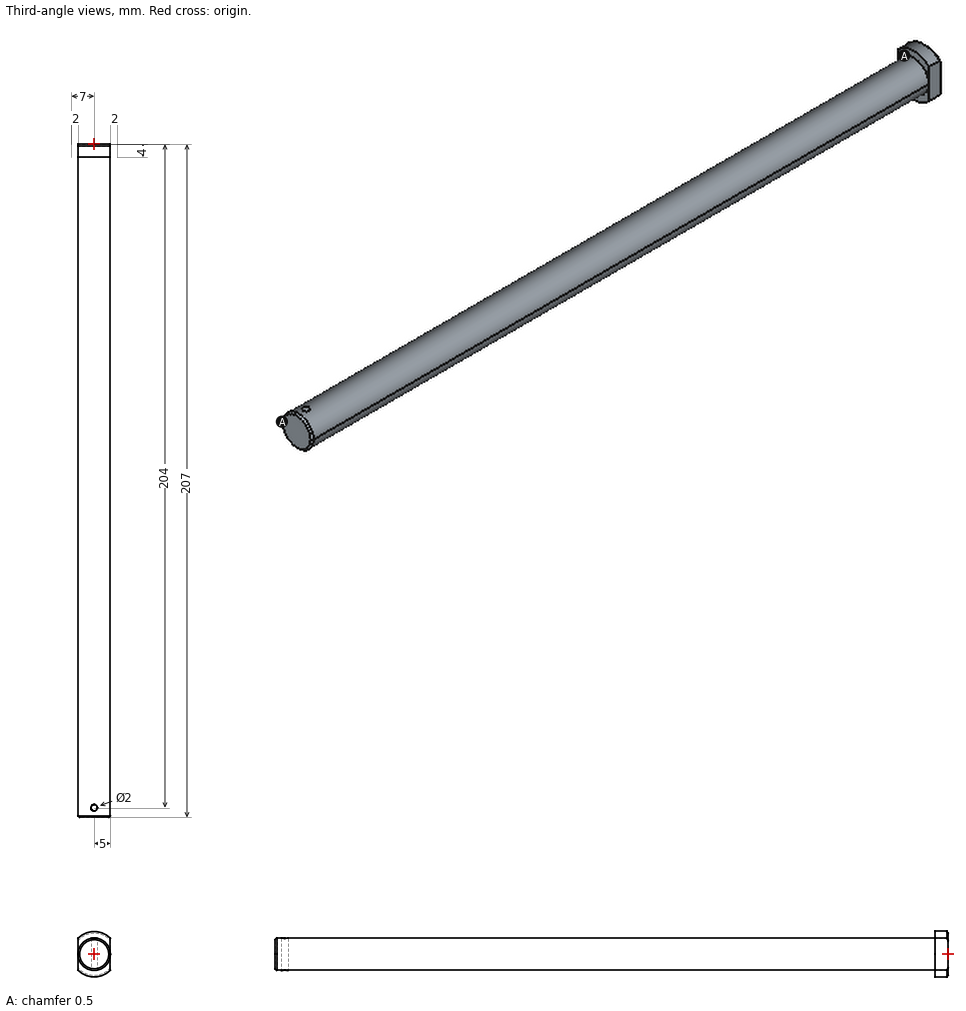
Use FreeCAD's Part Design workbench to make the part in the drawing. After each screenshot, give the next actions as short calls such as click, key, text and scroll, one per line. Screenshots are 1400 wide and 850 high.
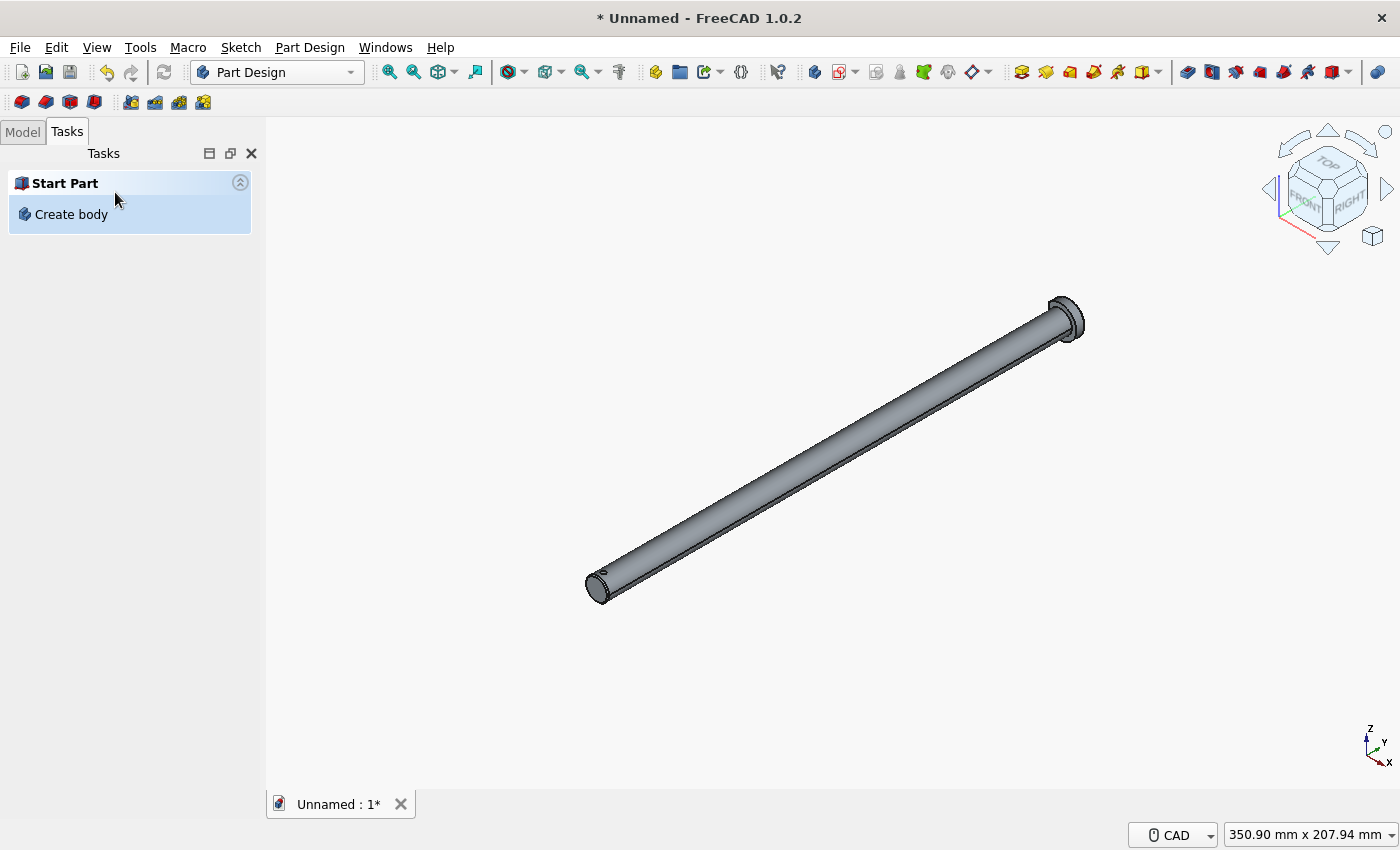
click(840, 72)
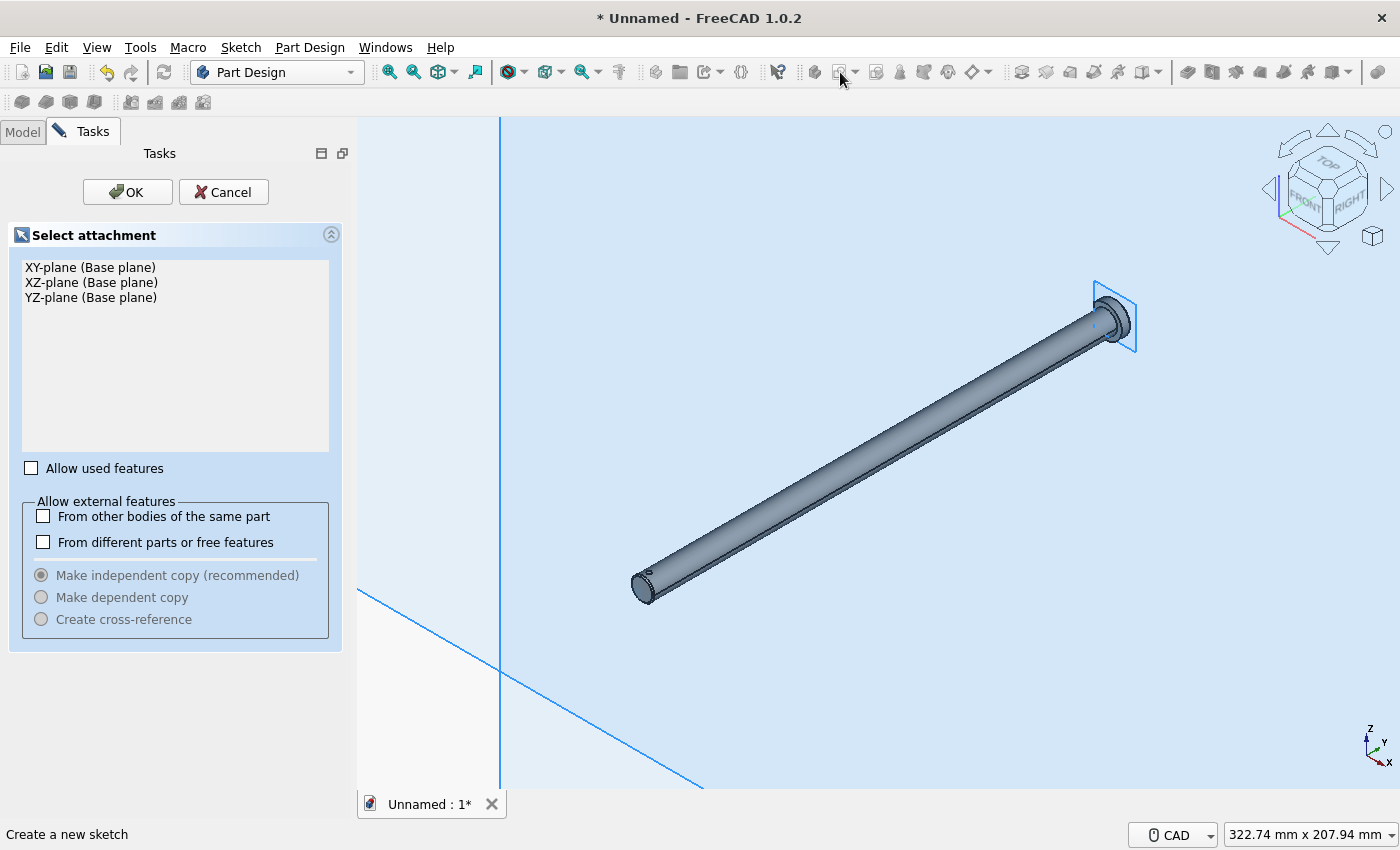
click(82, 268)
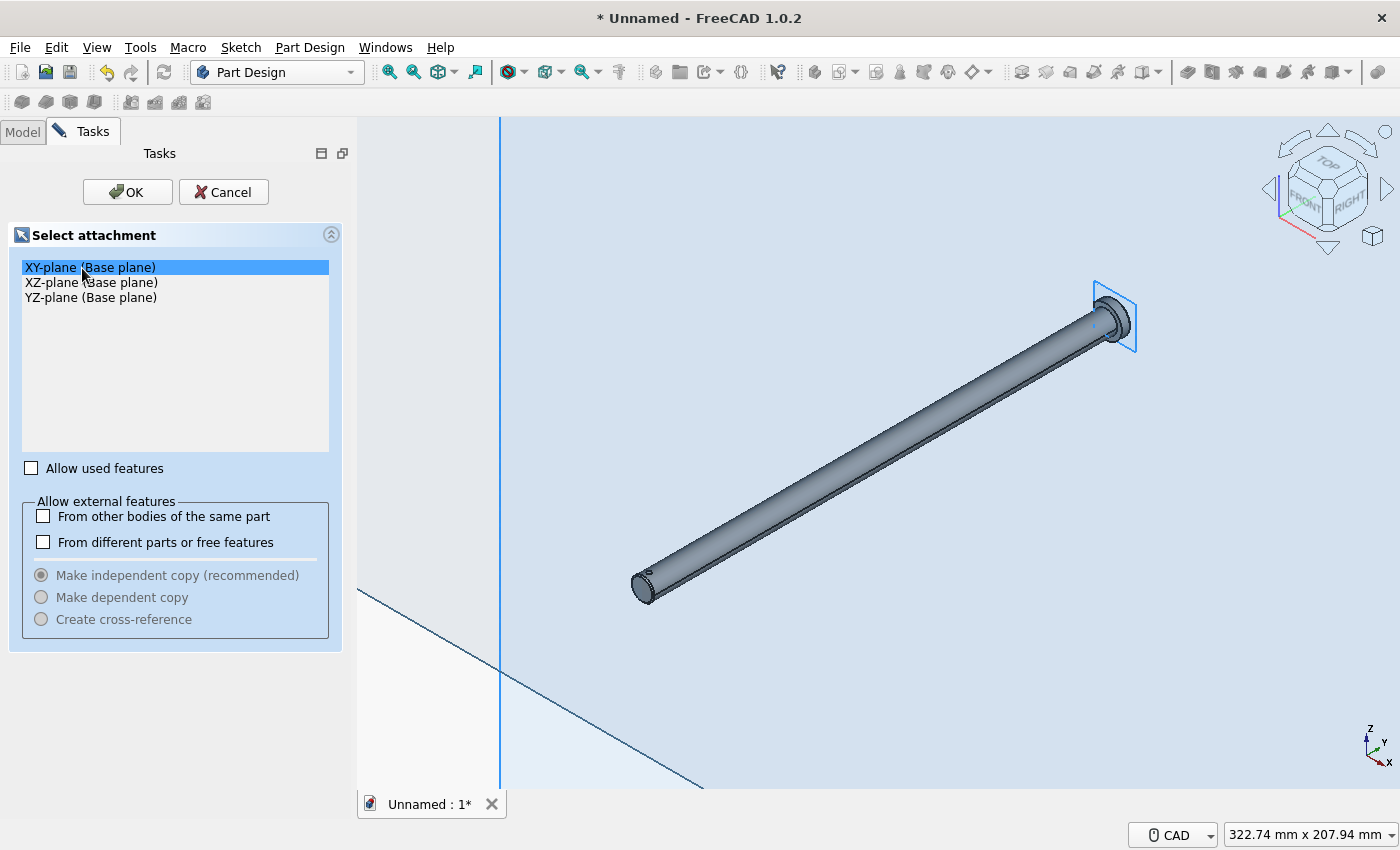
click(128, 192)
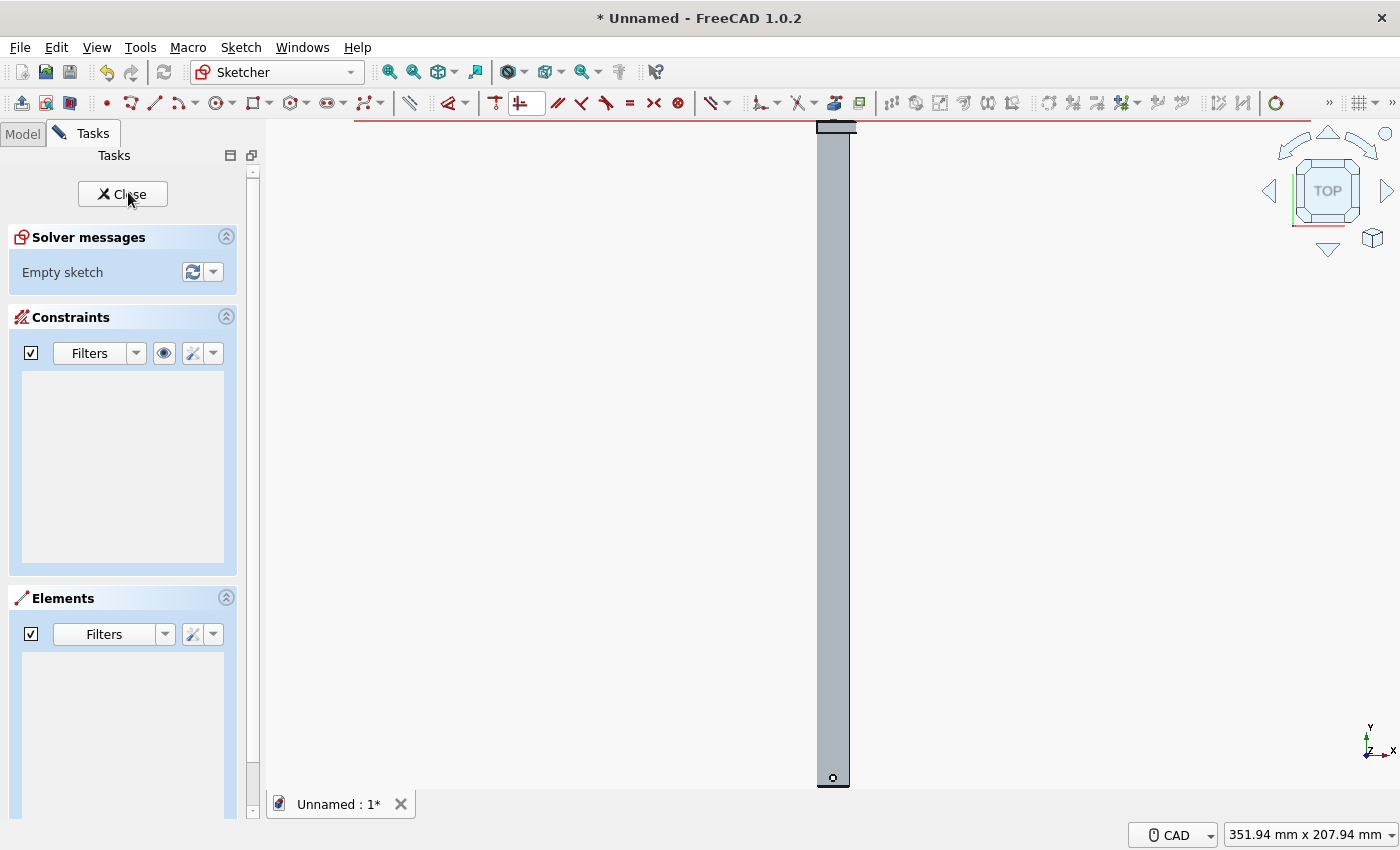
click(70, 104)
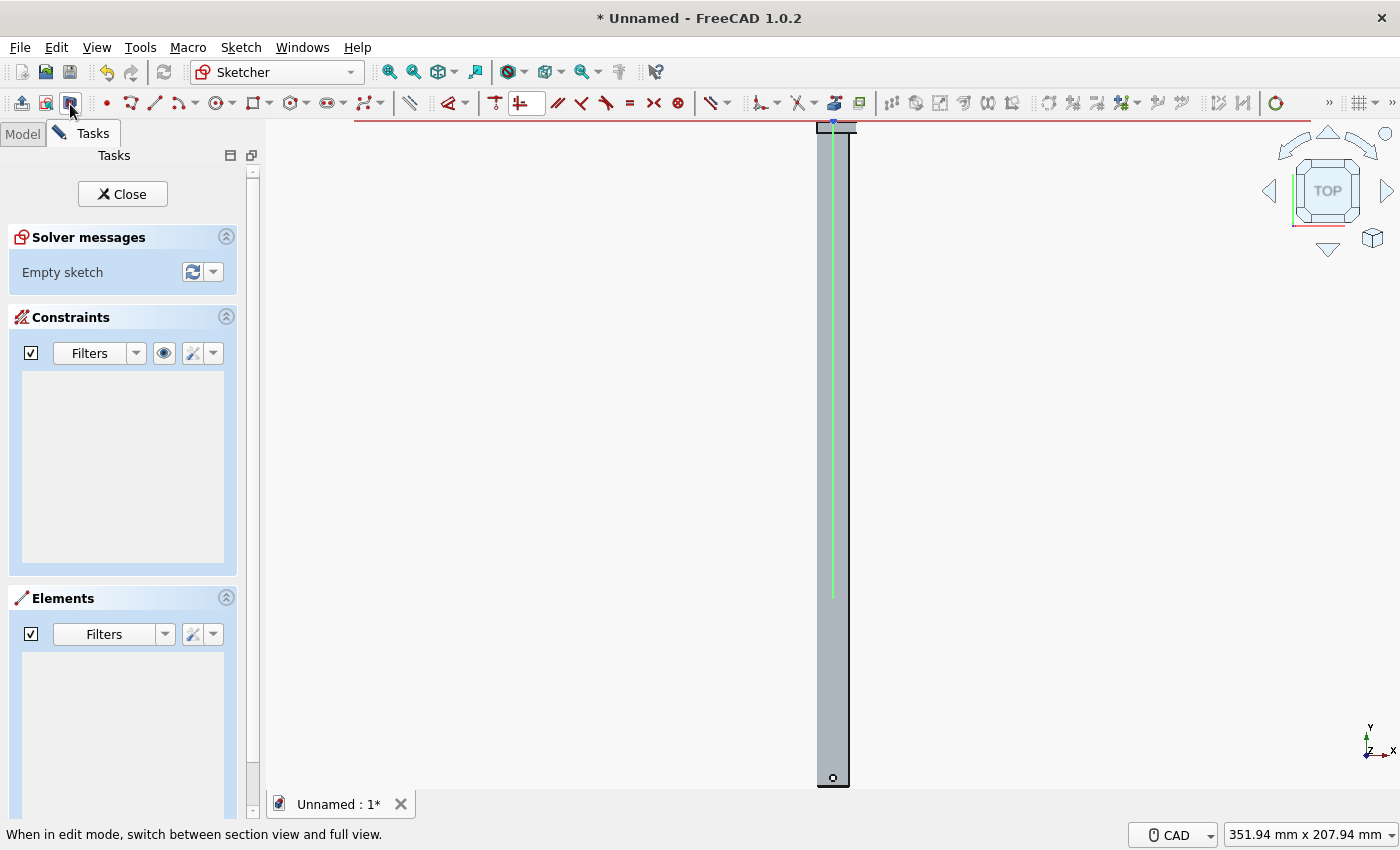
scroll(764, 454, down, 5)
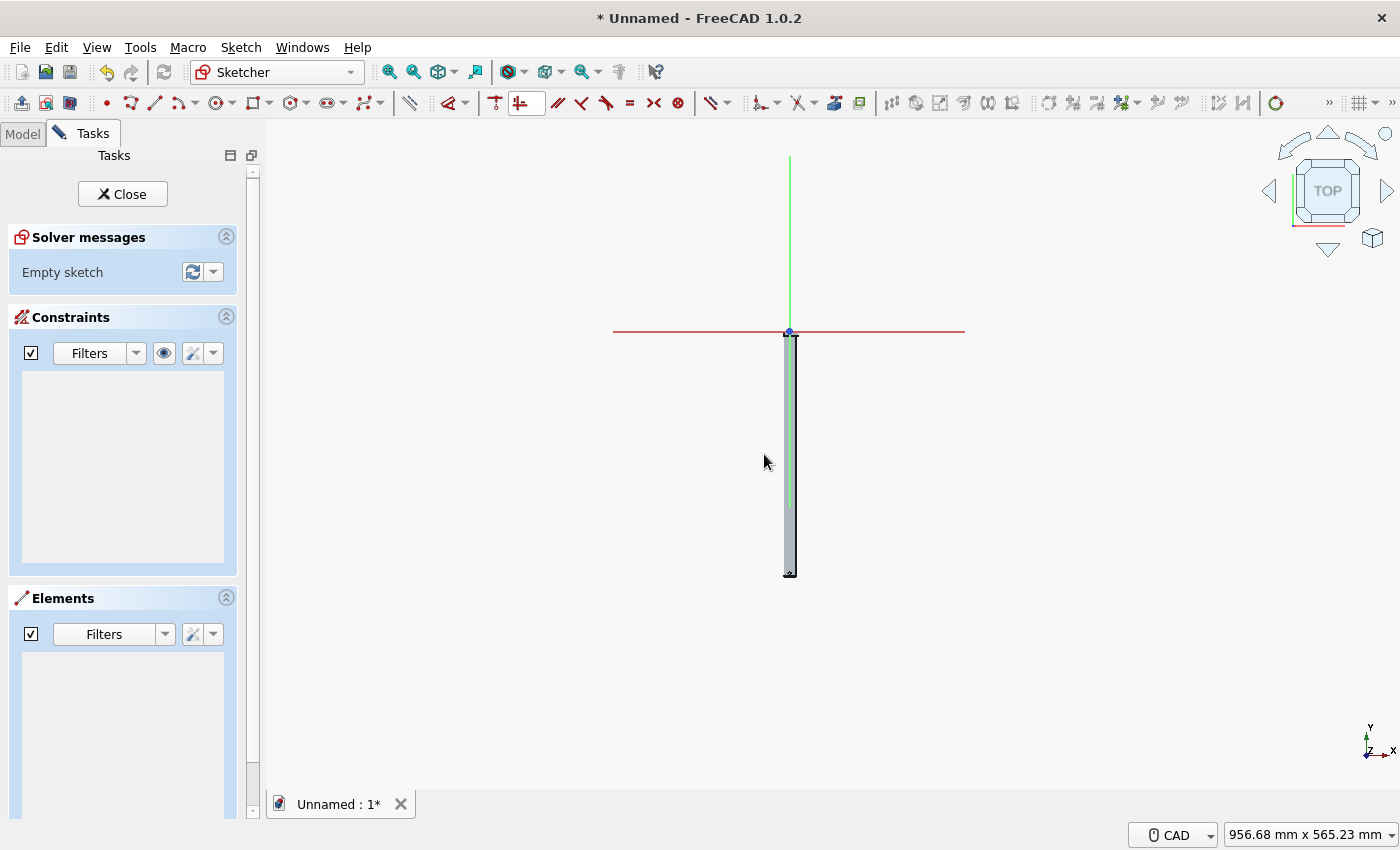
scroll(795, 328, up, 15)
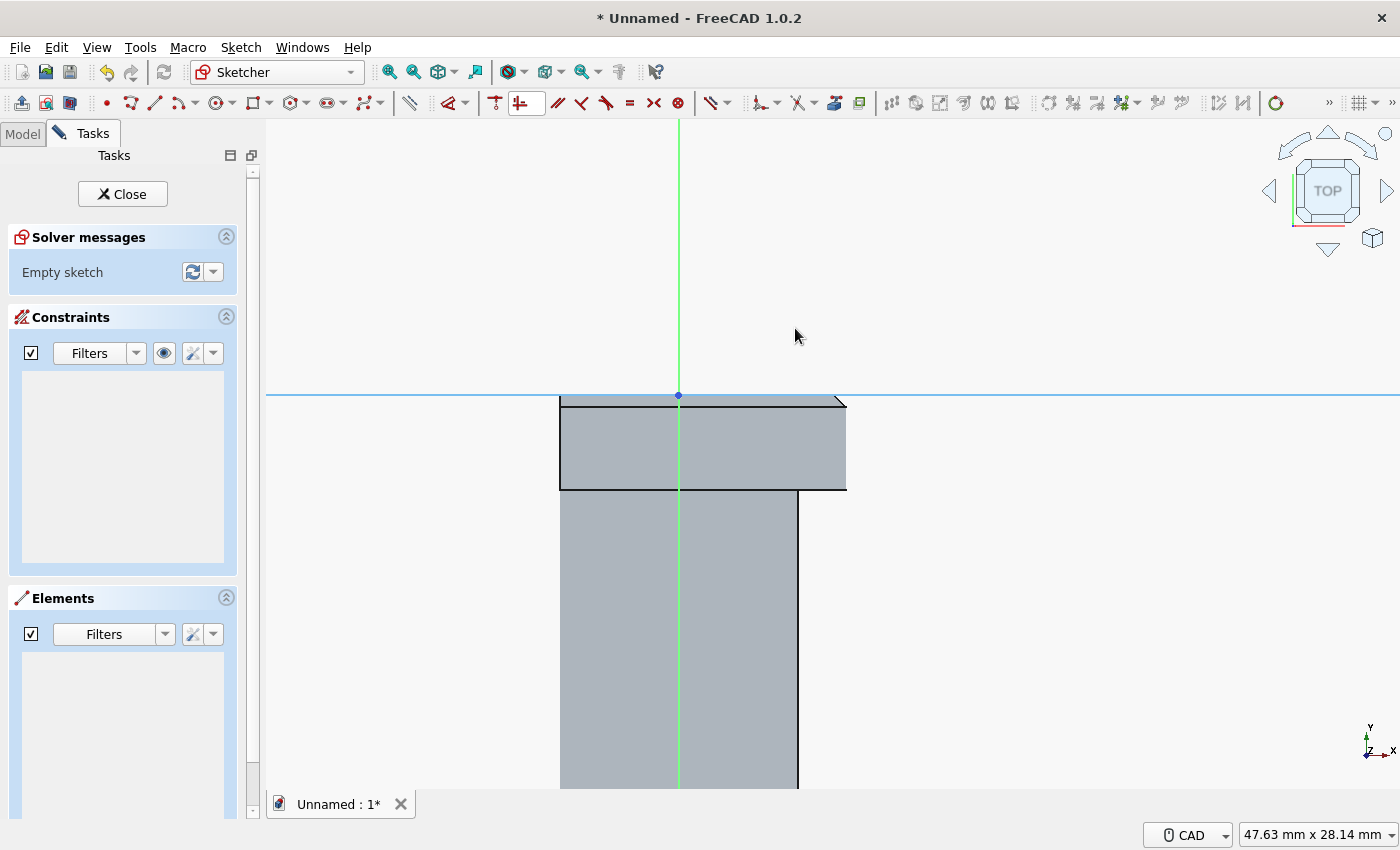
scroll(761, 439, up, 7)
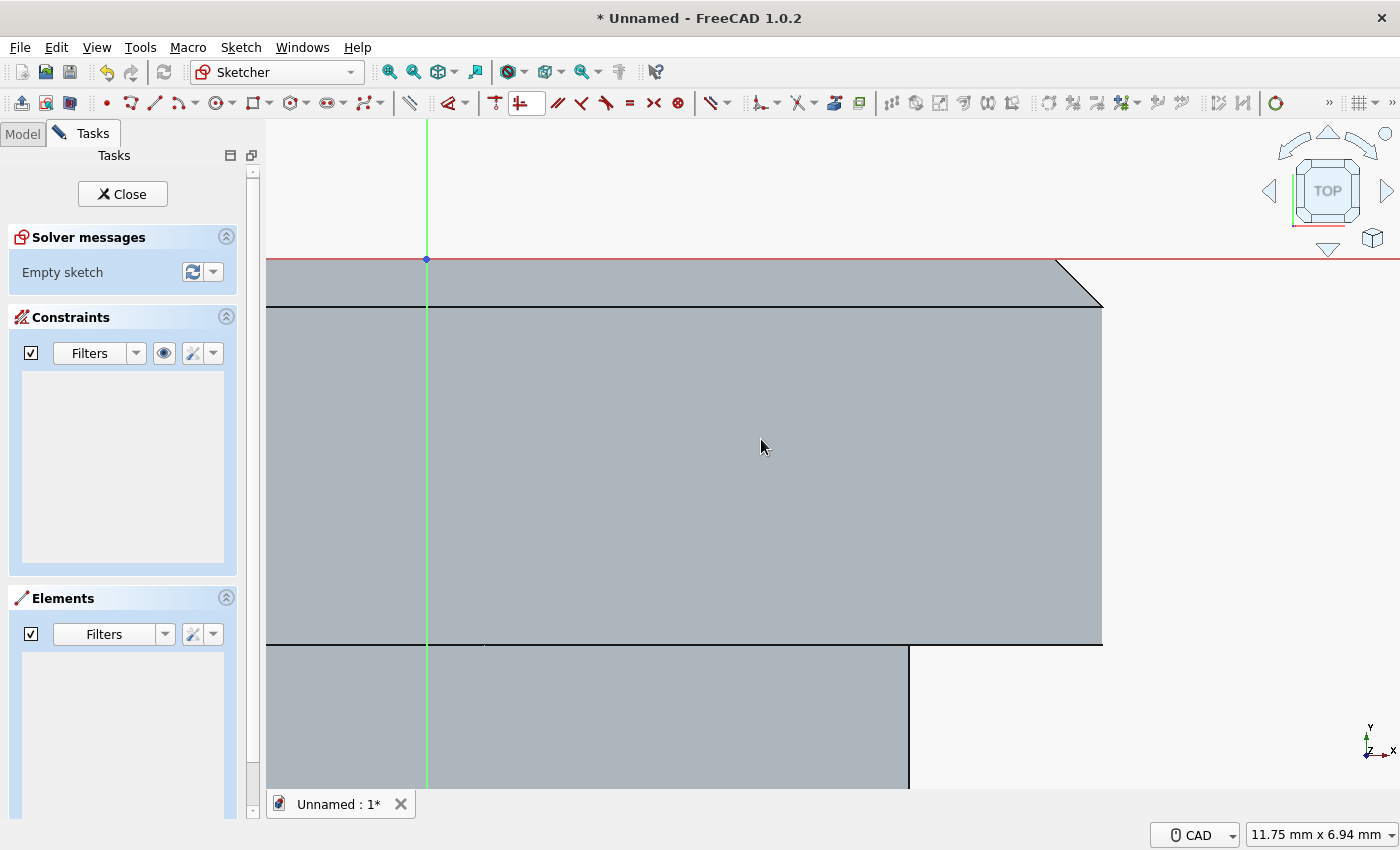
click(254, 104)